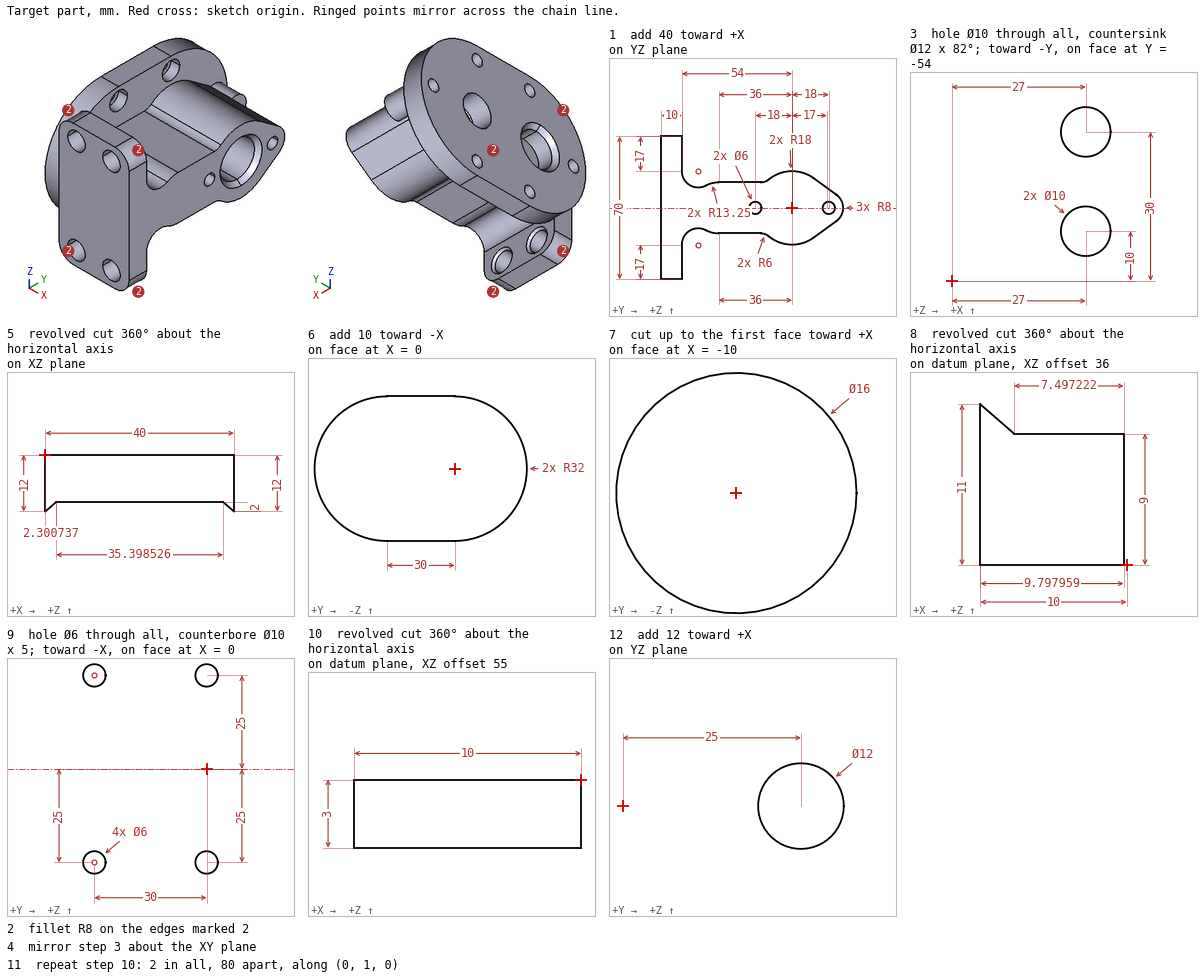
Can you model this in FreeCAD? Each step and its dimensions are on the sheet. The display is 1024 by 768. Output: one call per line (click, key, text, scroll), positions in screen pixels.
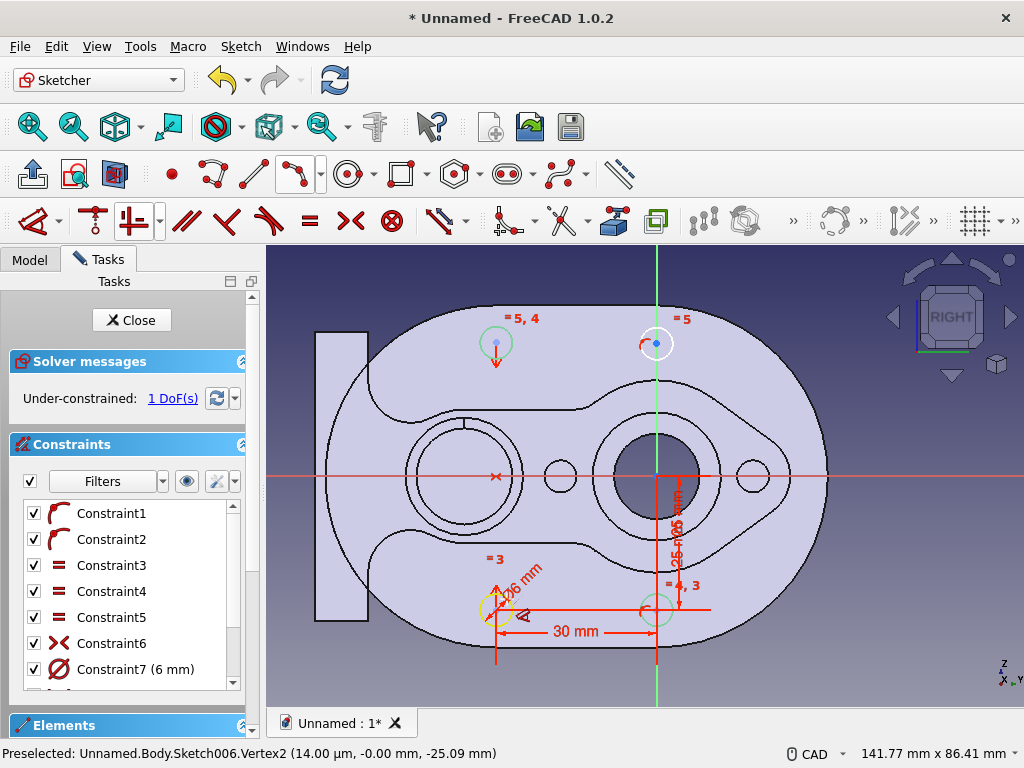
click(657, 344)
click(691, 410)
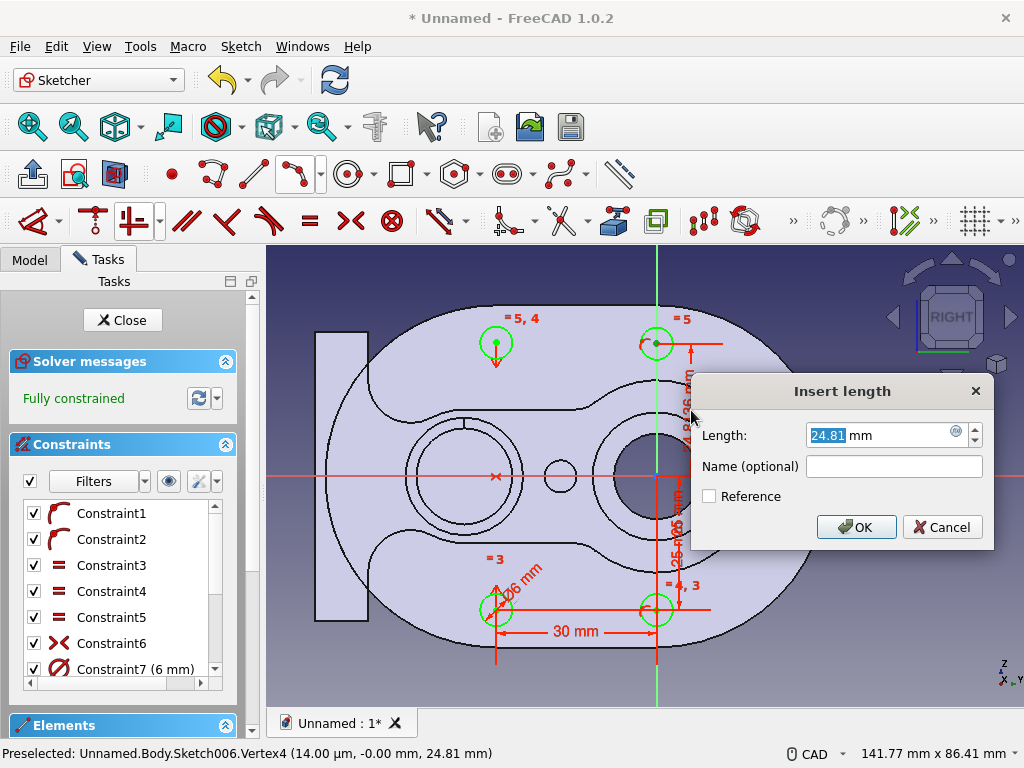
text(25)
key(Return)
key(Escape)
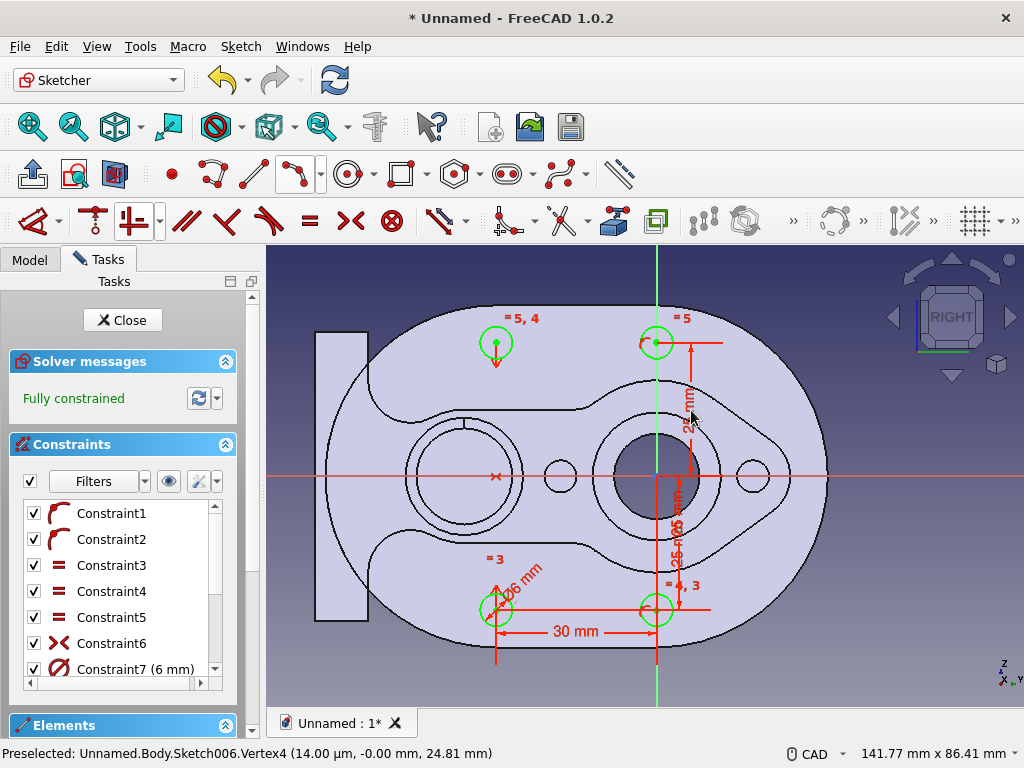
click(123, 320)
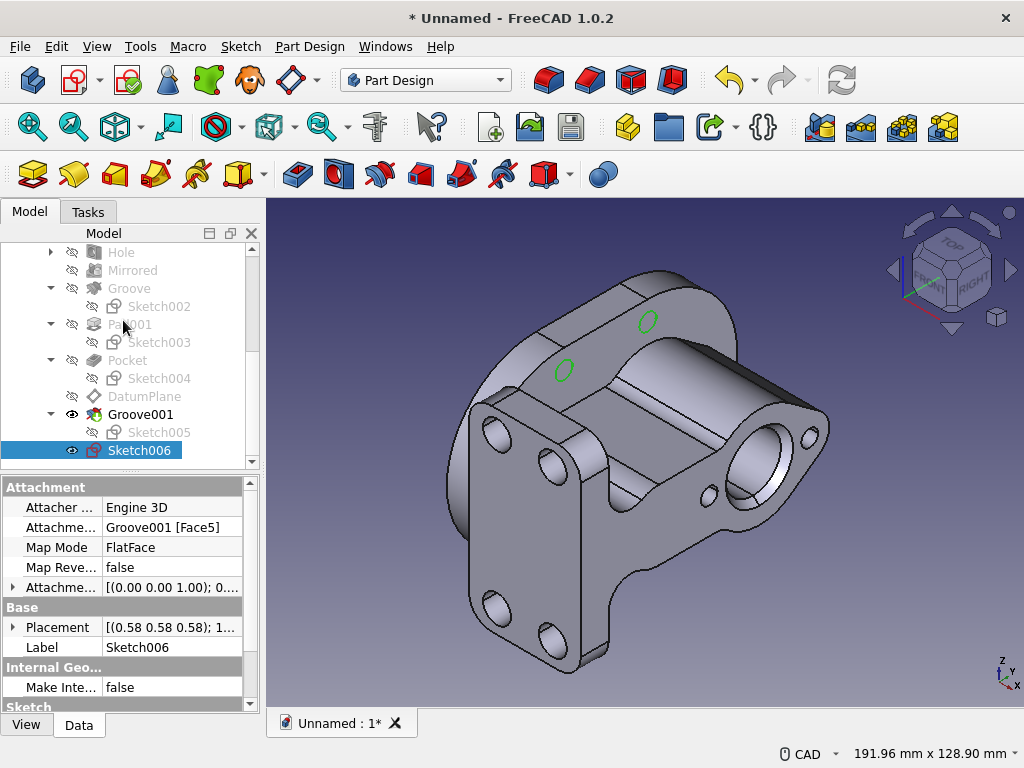
click(339, 174)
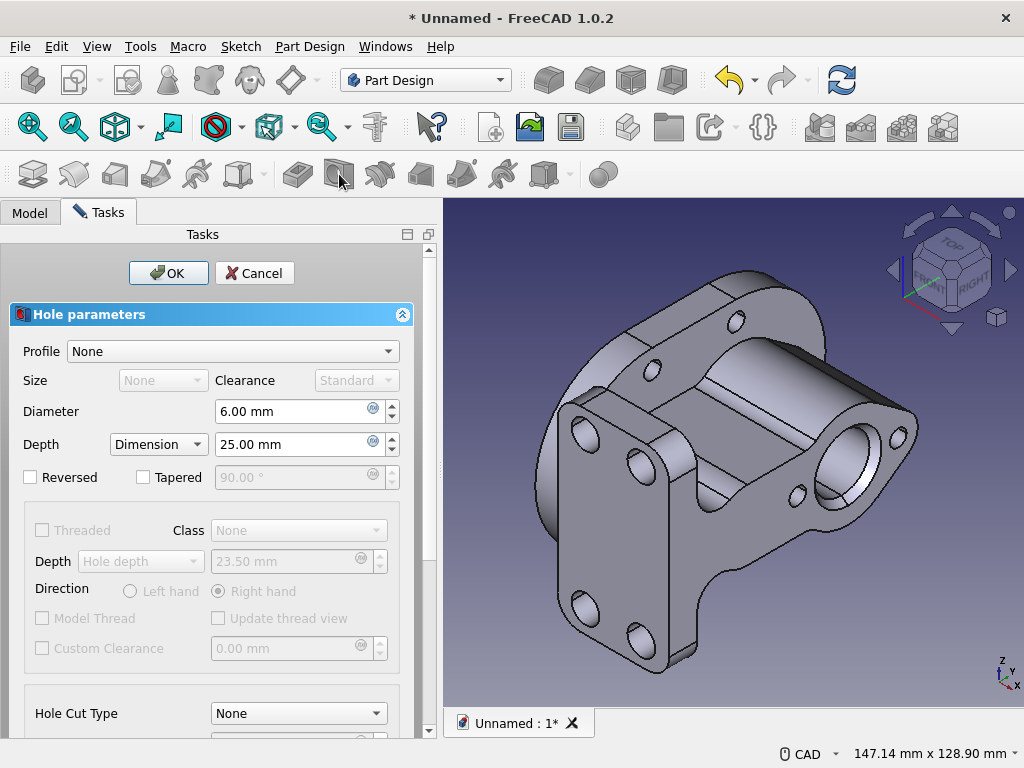
triple_click(300, 412)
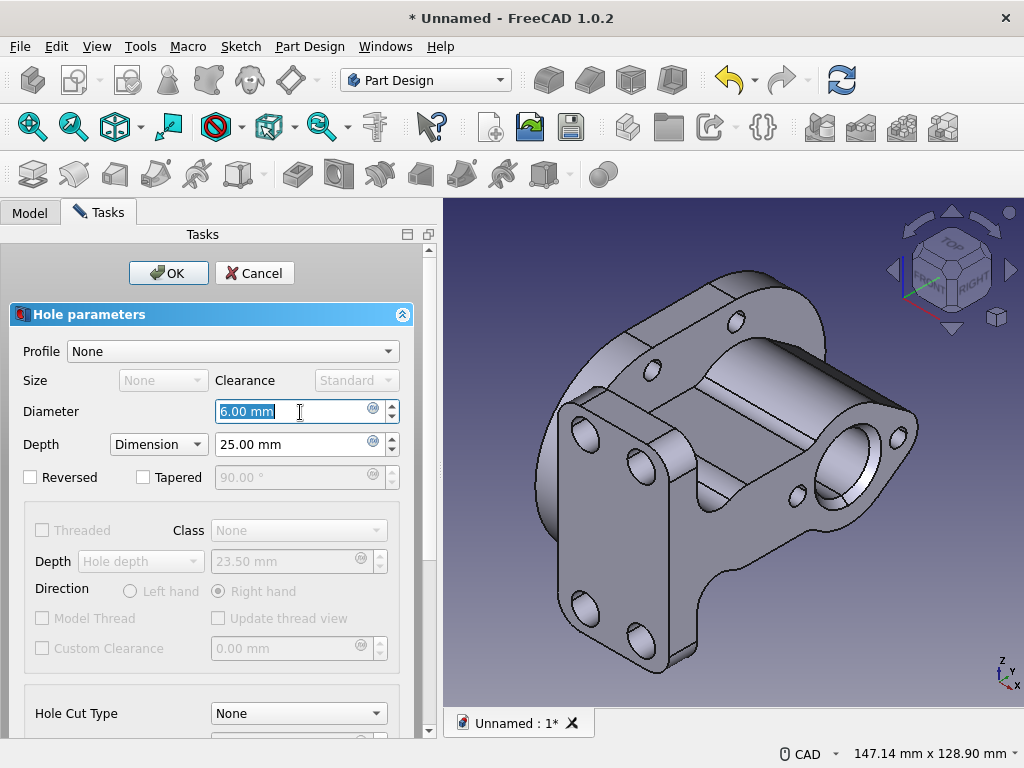
text(6)
key(Tab)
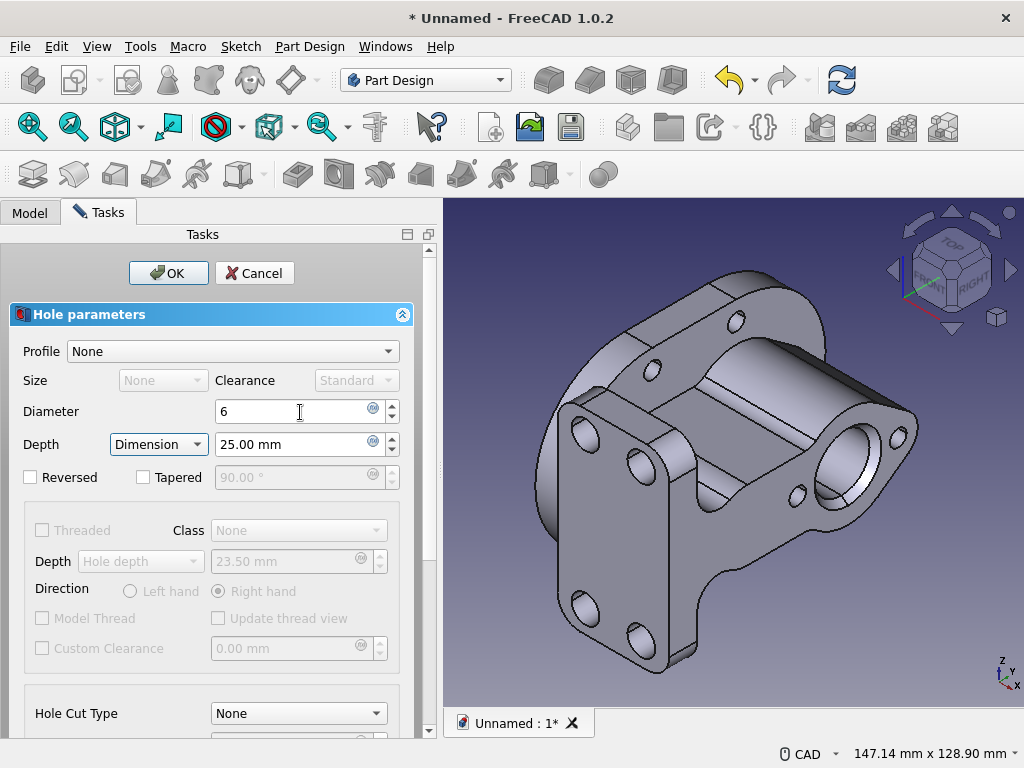
click(160, 444)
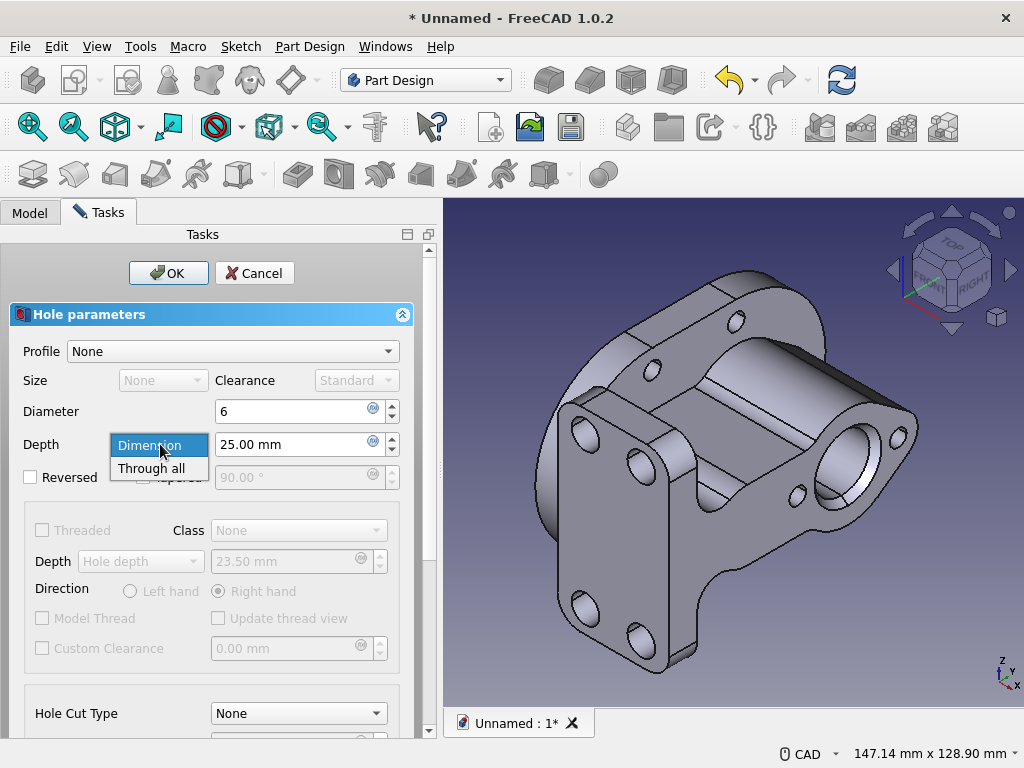
click(158, 468)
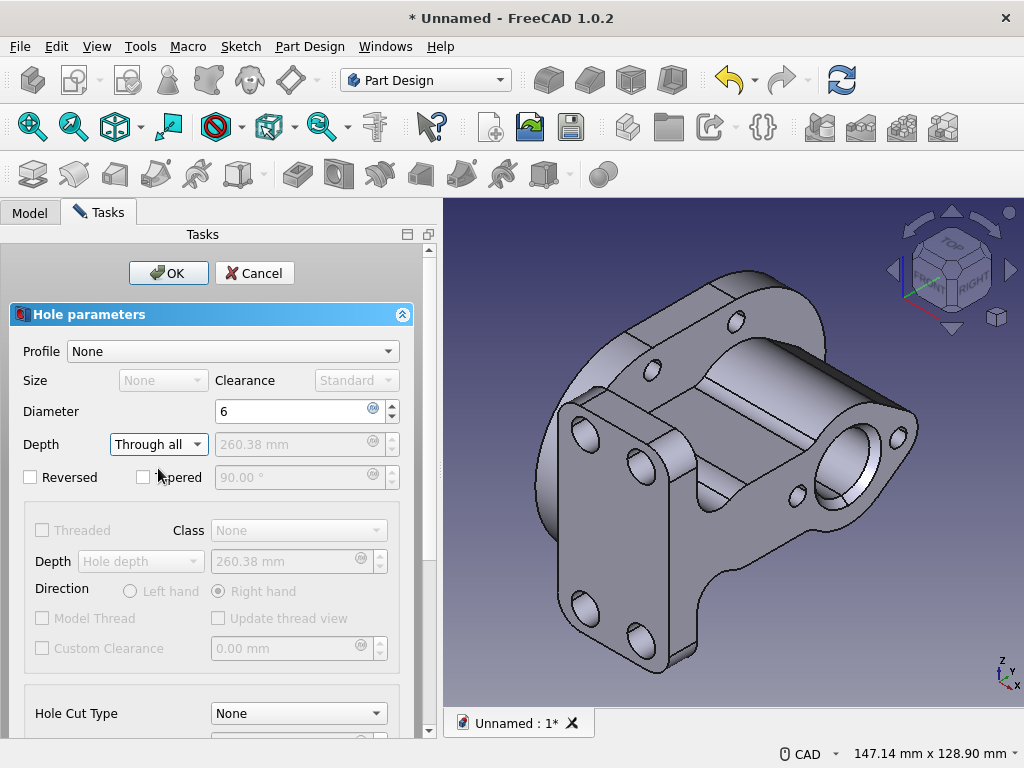
click(300, 714)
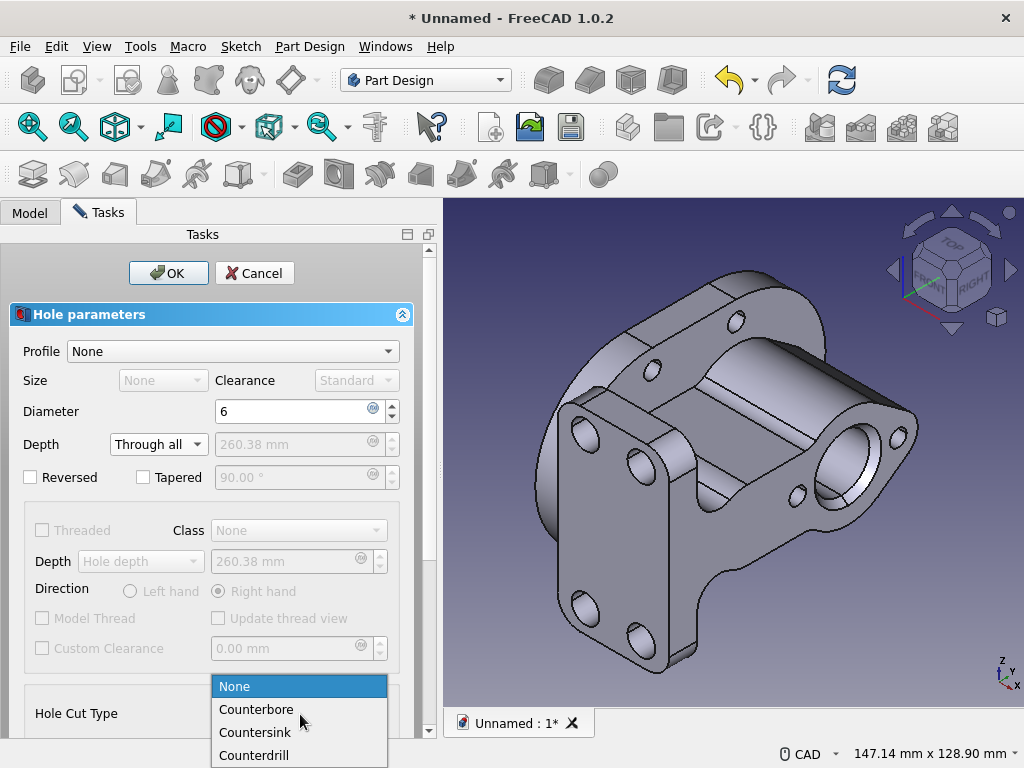
click(298, 710)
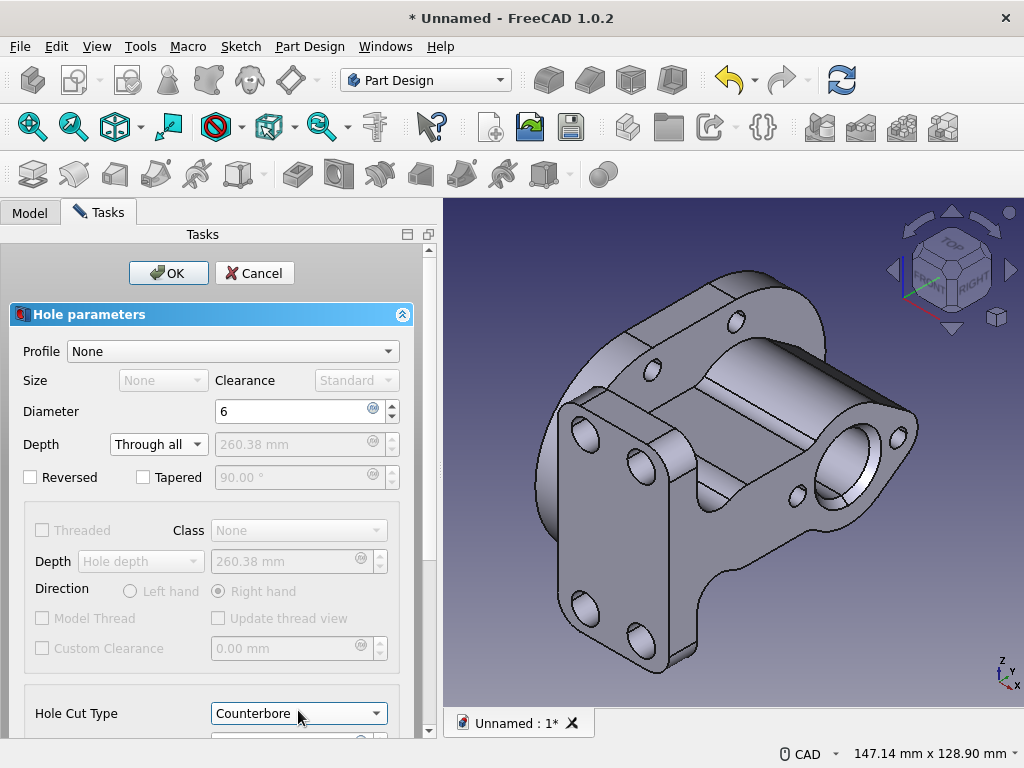
scroll(429, 491, down, 2)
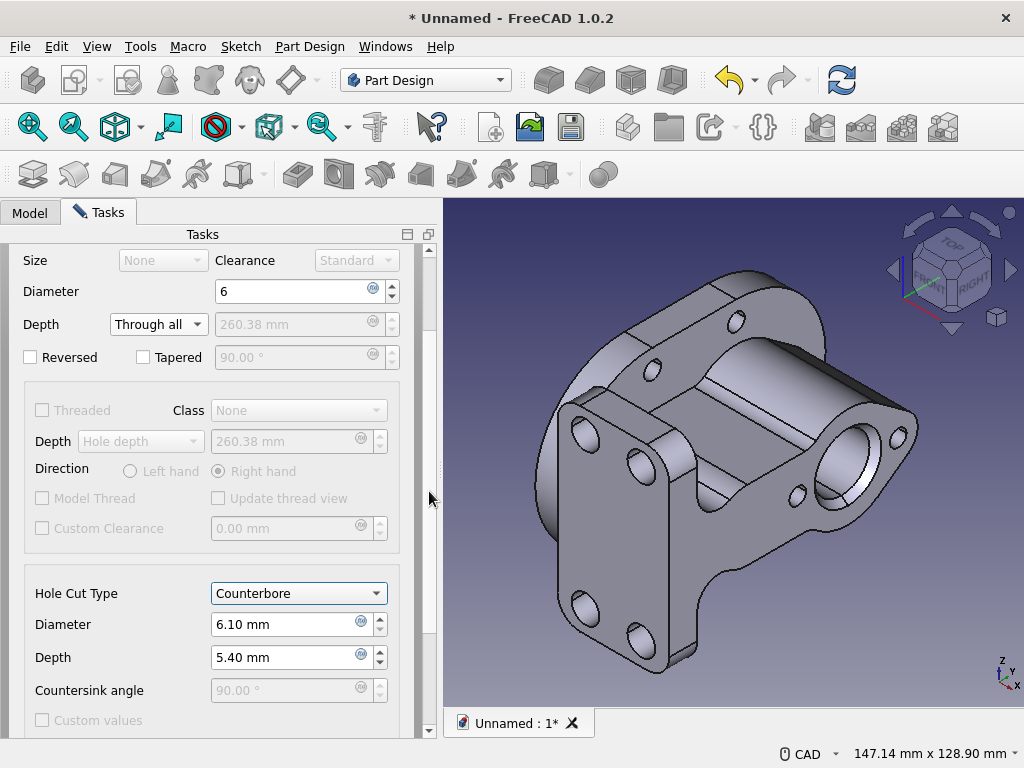
triple_click(292, 624)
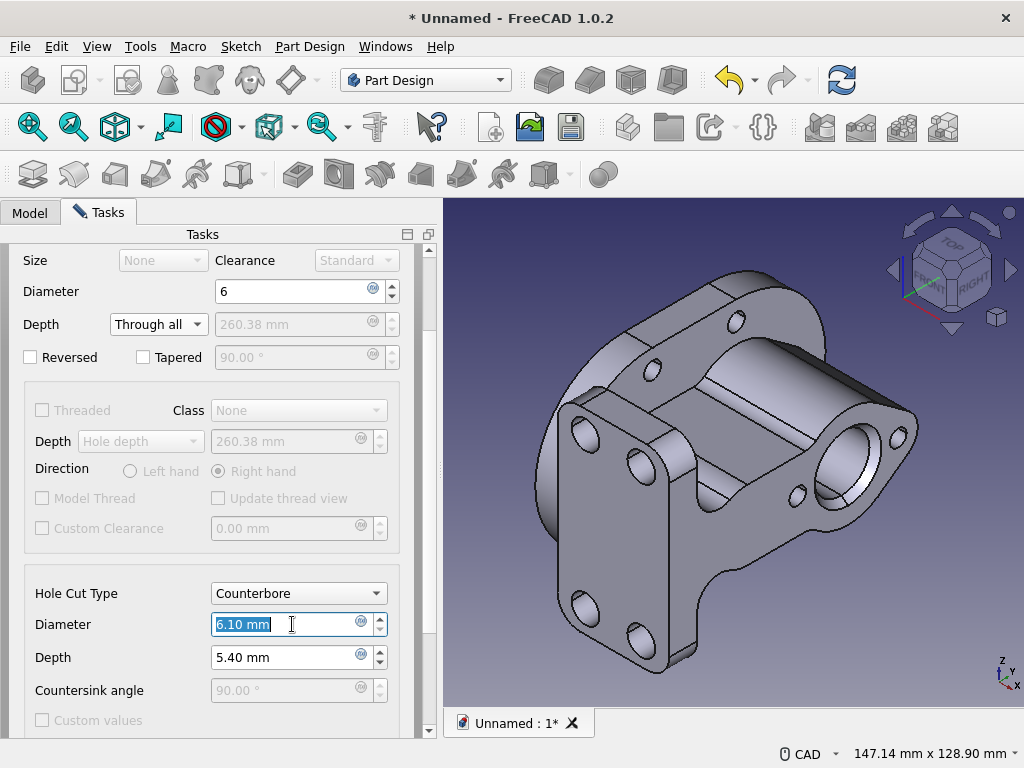
text(10)
key(Tab)